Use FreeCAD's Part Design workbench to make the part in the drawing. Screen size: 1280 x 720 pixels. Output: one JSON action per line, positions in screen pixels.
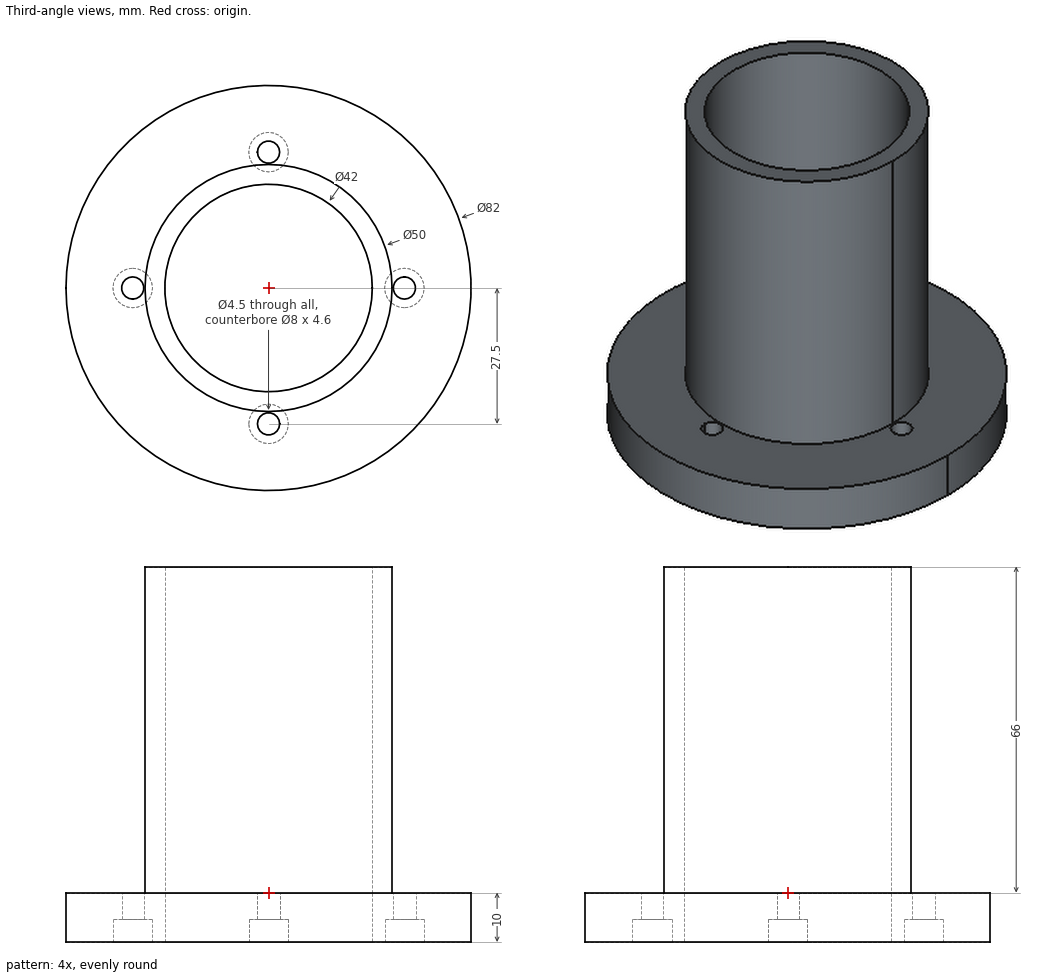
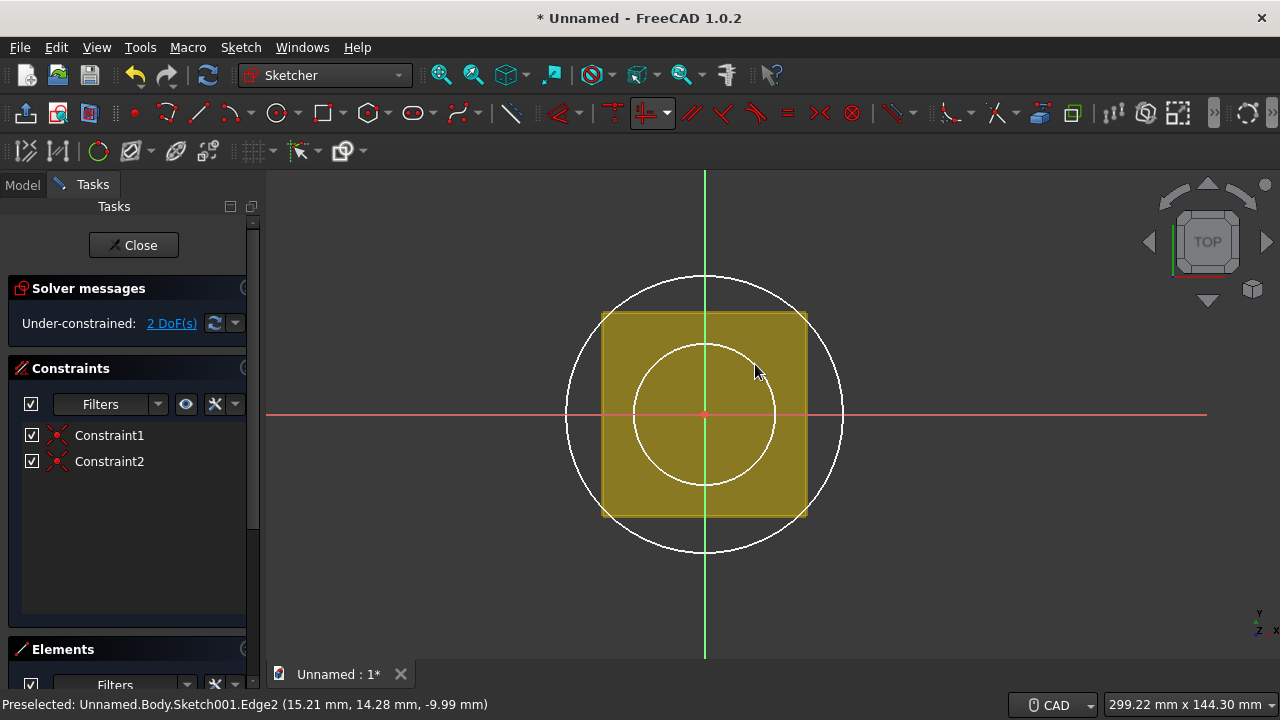
{"action": "left_click", "coordinate": [558, 114]}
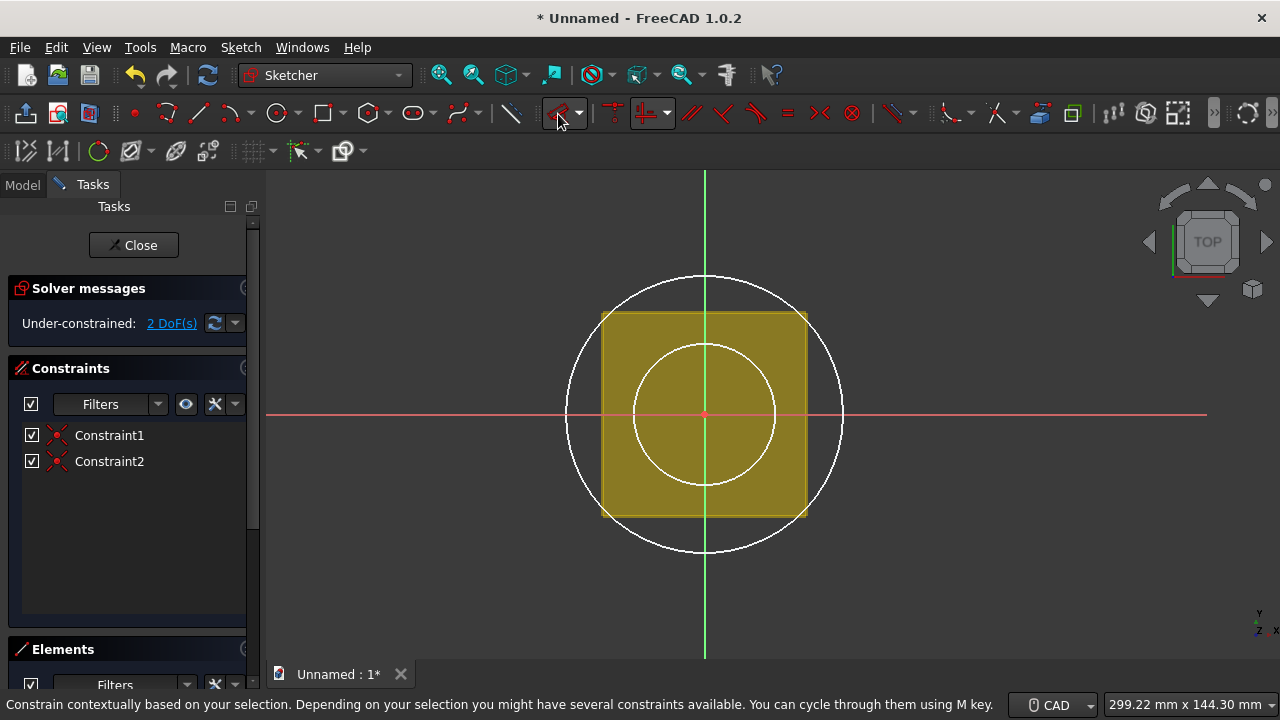
{"action": "left_click", "coordinate": [802, 316]}
{"action": "left_click", "coordinate": [825, 293]}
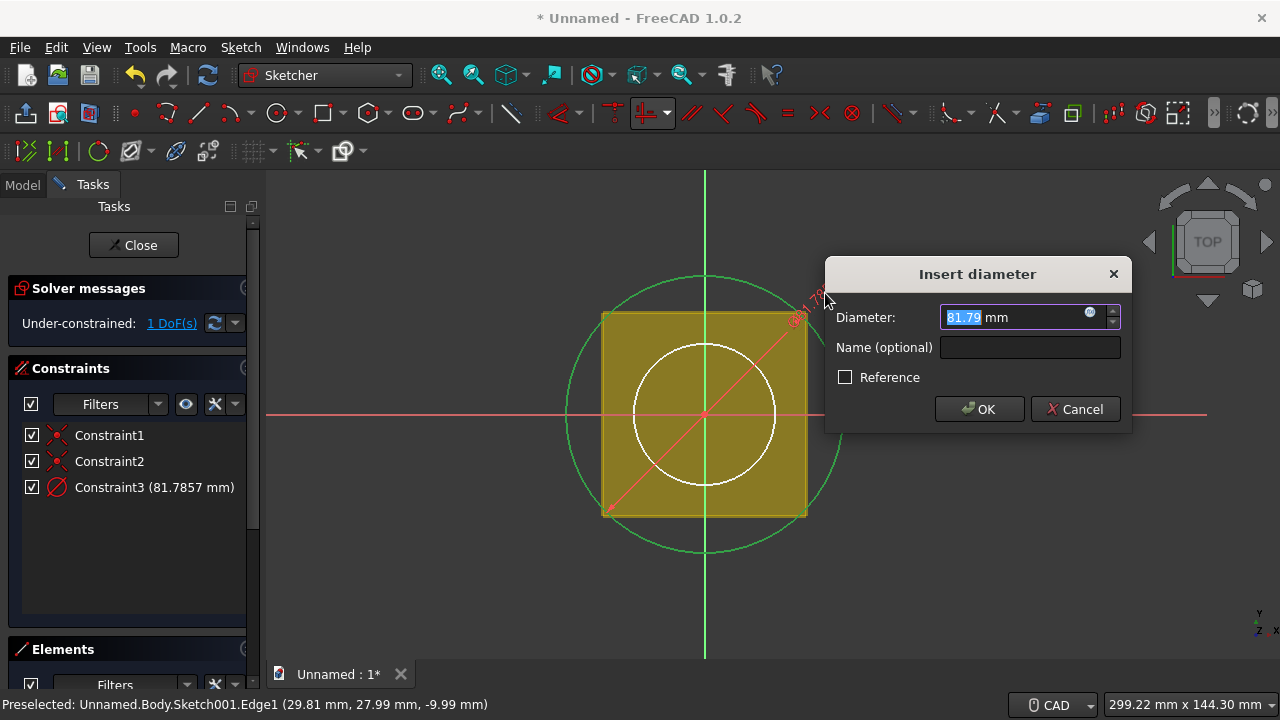
{"action": "type", "text": "82"}
{"action": "key", "text": "Return"}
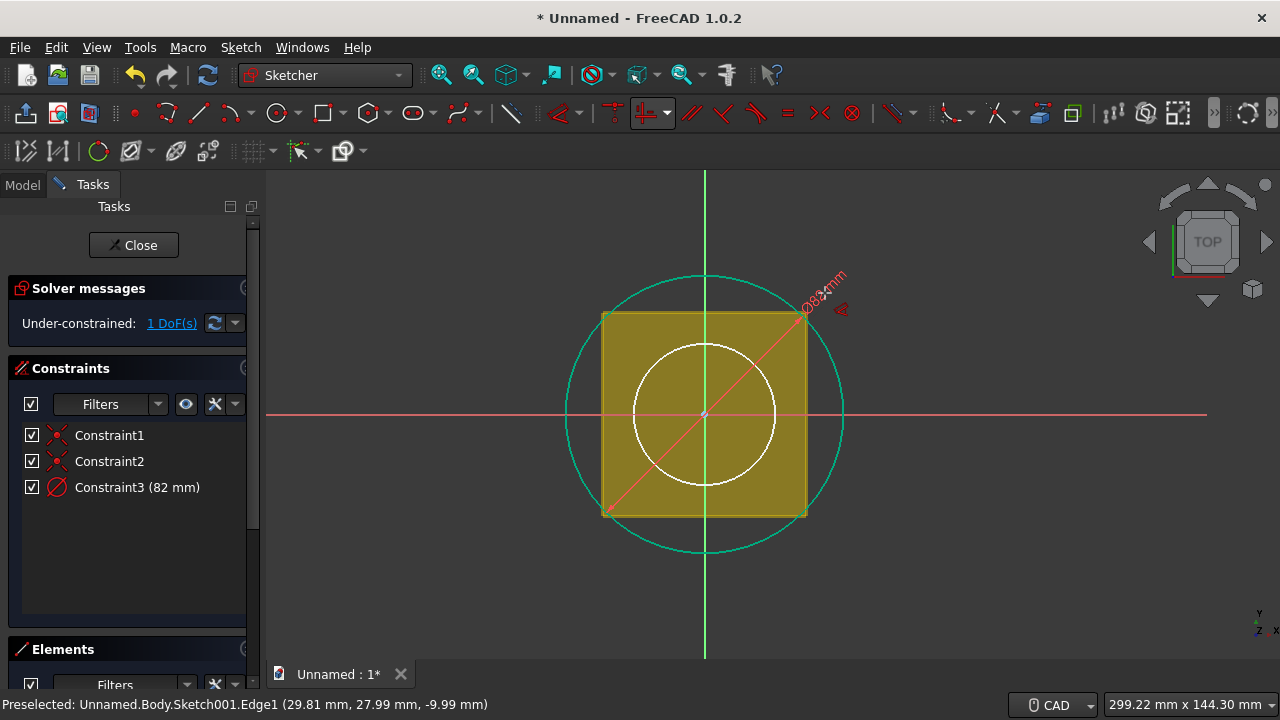
{"action": "left_click", "coordinate": [754, 364]}
{"action": "left_click", "coordinate": [776, 341]}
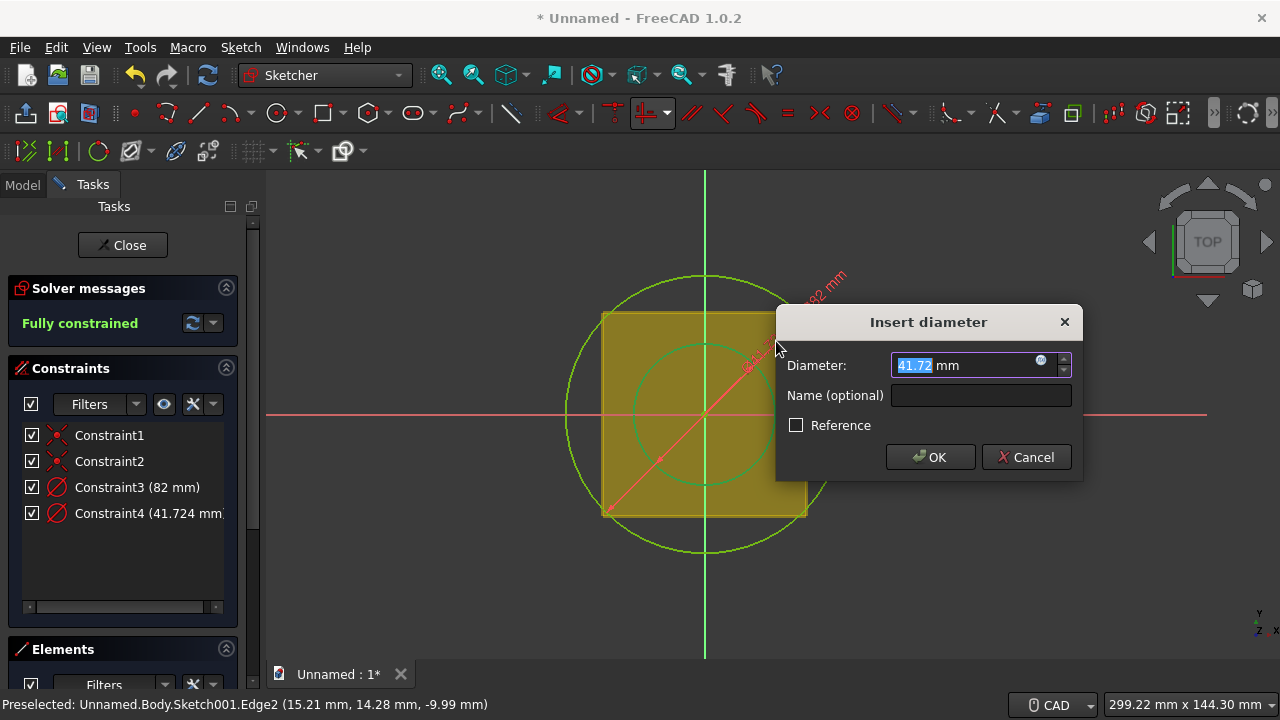
{"action": "type", "text": "42"}
{"action": "key", "text": "Return"}
{"action": "key", "text": "Escape"}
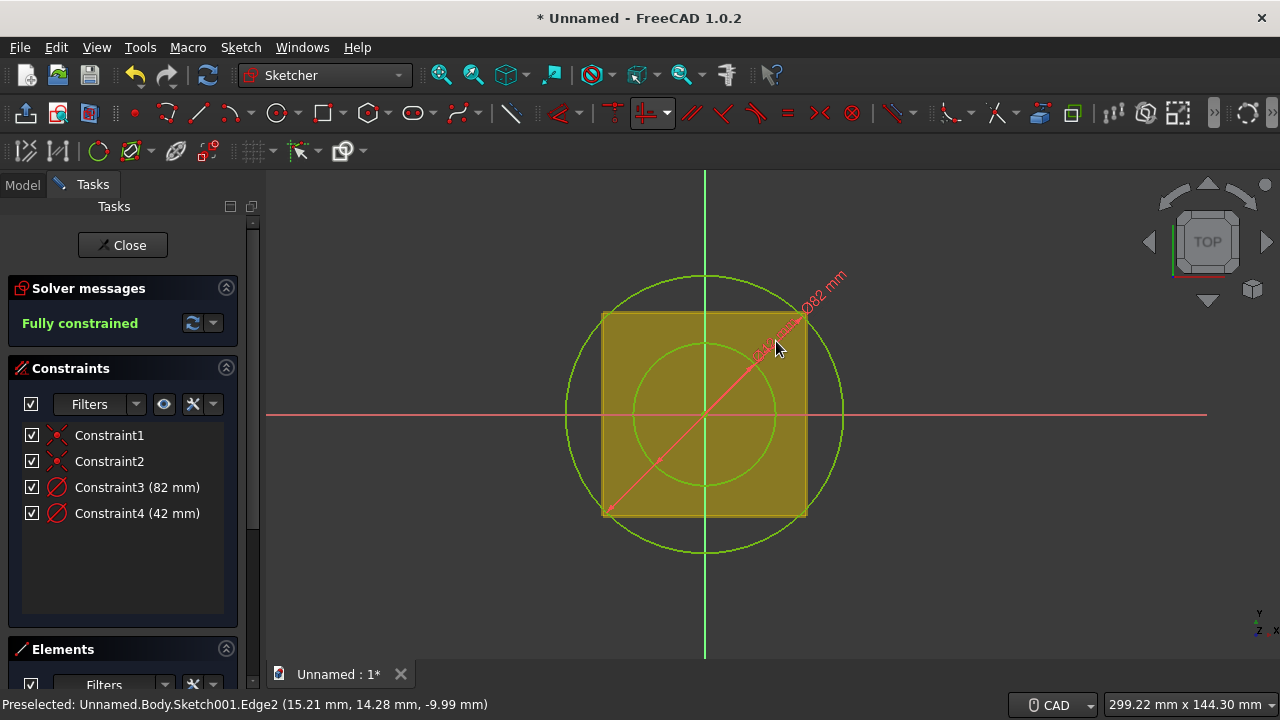
{"action": "left_click", "coordinate": [123, 245]}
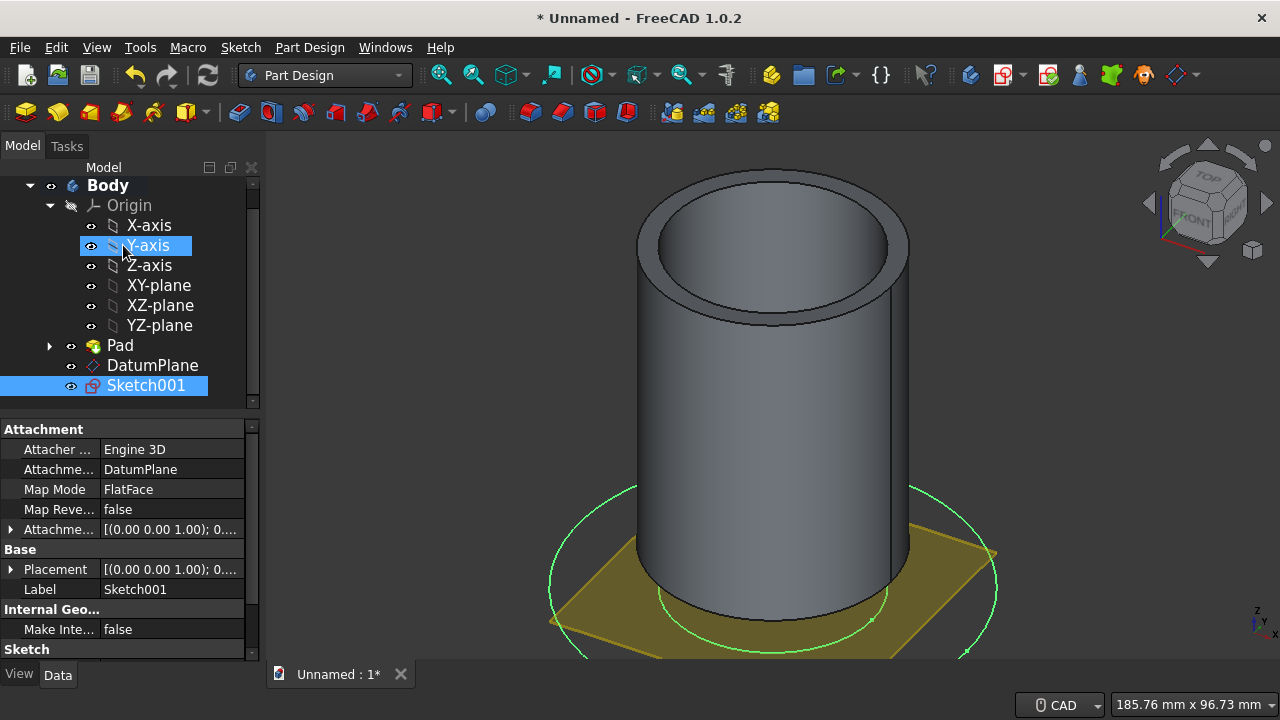
{"action": "left_click", "coordinate": [26, 112]}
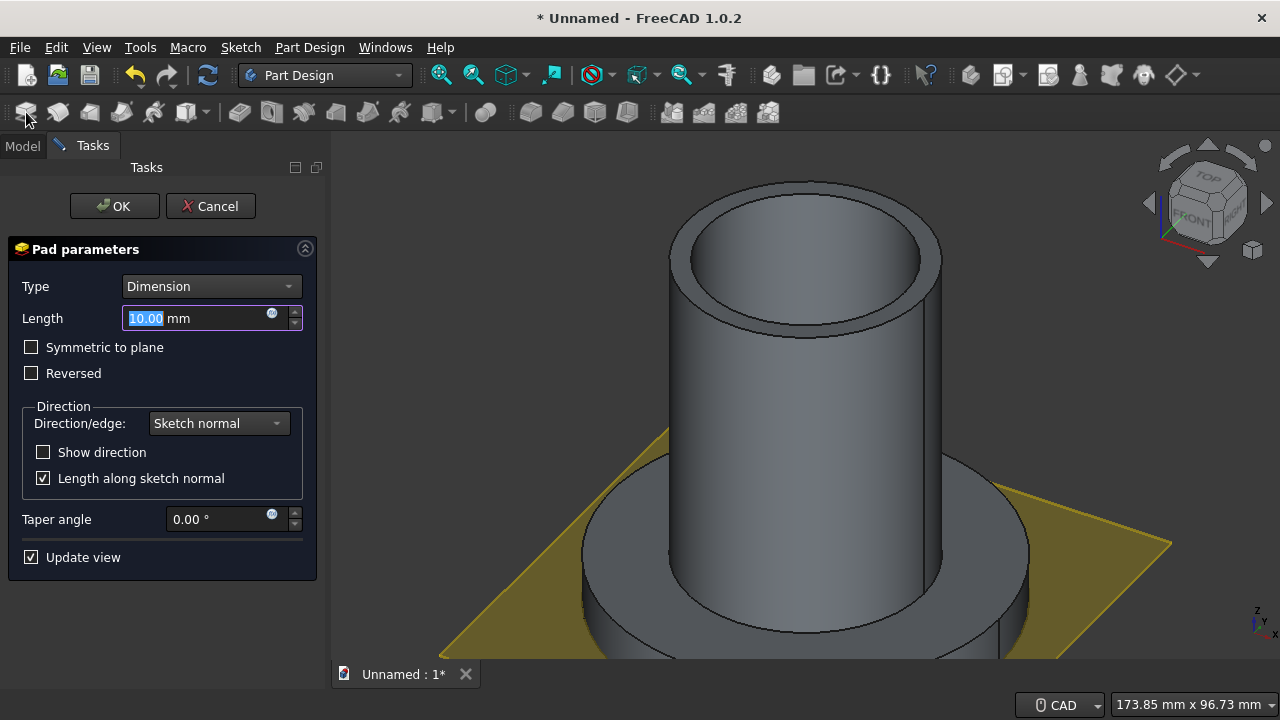
{"action": "type", "text": "10"}
{"action": "key", "text": "Tab"}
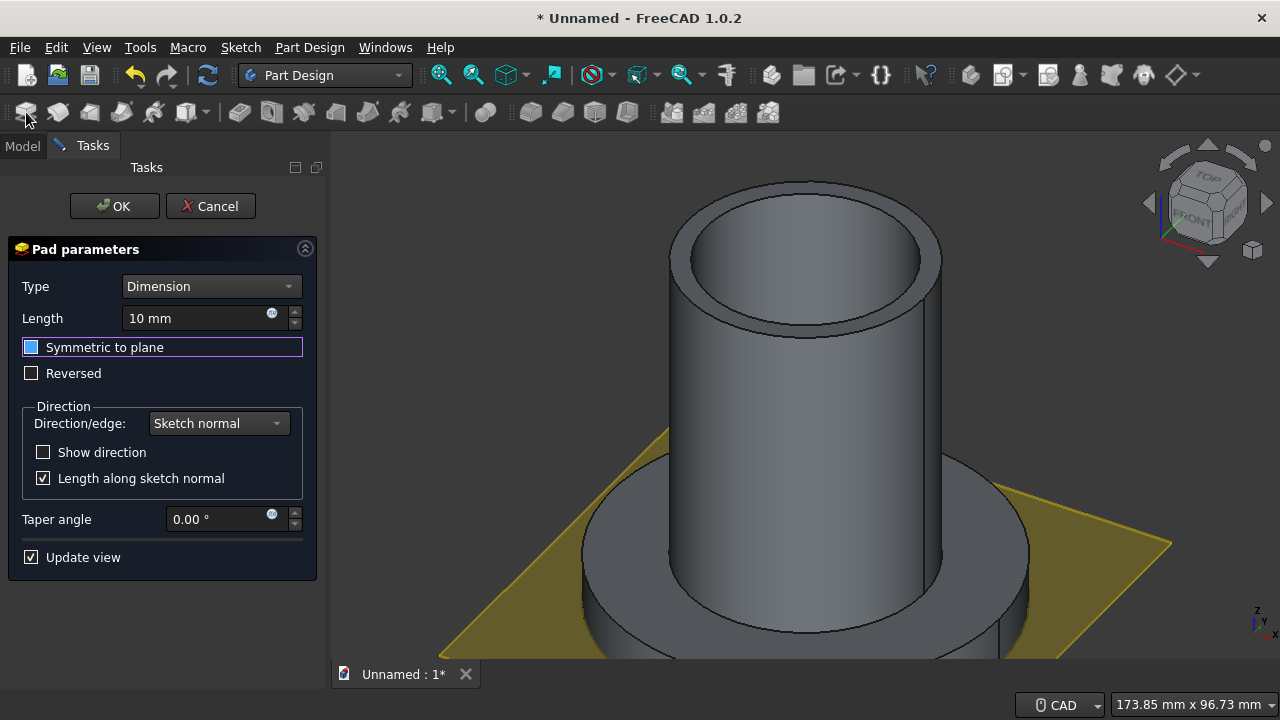
{"action": "left_click", "coordinate": [115, 206]}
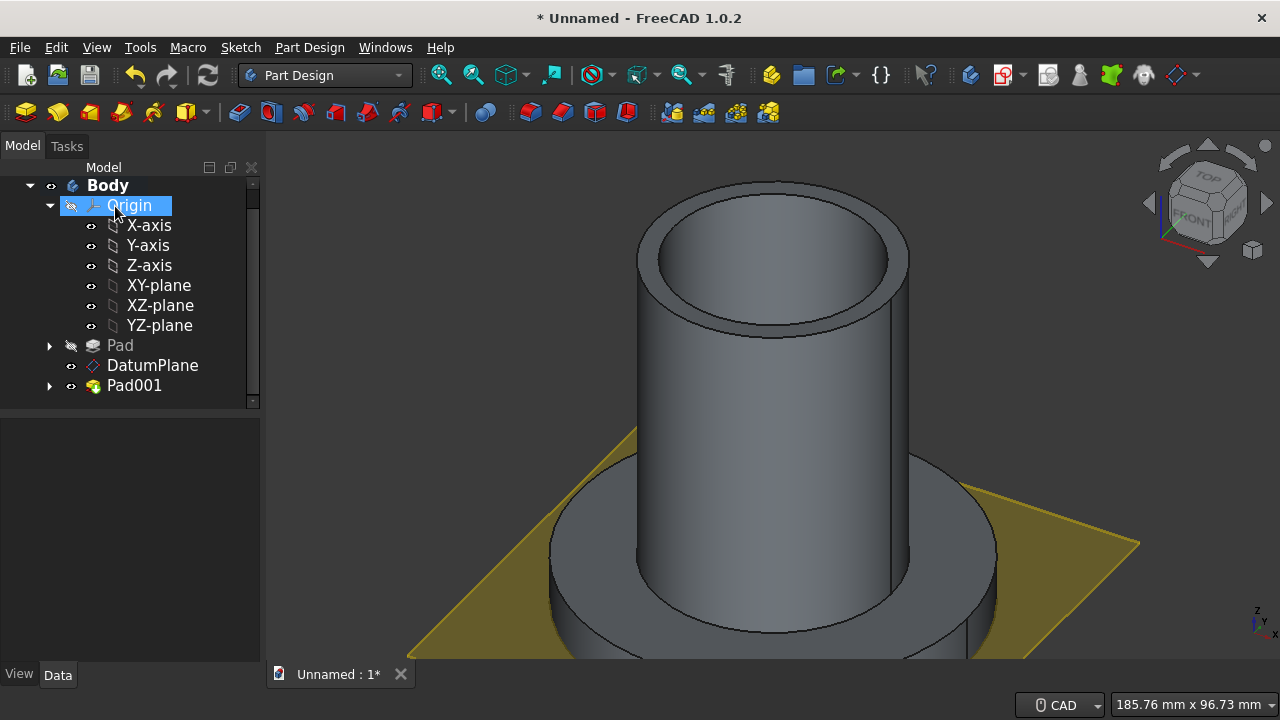
{"action": "left_click", "coordinate": [116, 366]}
{"action": "key", "text": "space"}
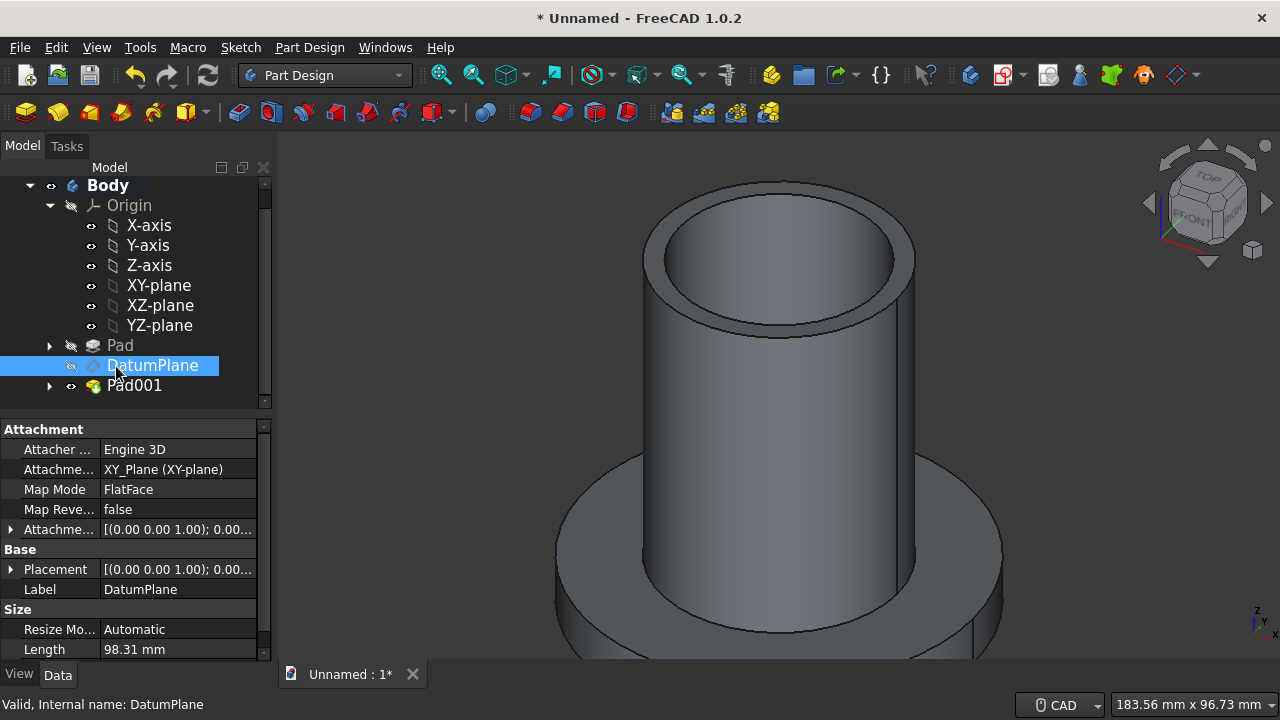
{"action": "left_click", "coordinate": [442, 76]}